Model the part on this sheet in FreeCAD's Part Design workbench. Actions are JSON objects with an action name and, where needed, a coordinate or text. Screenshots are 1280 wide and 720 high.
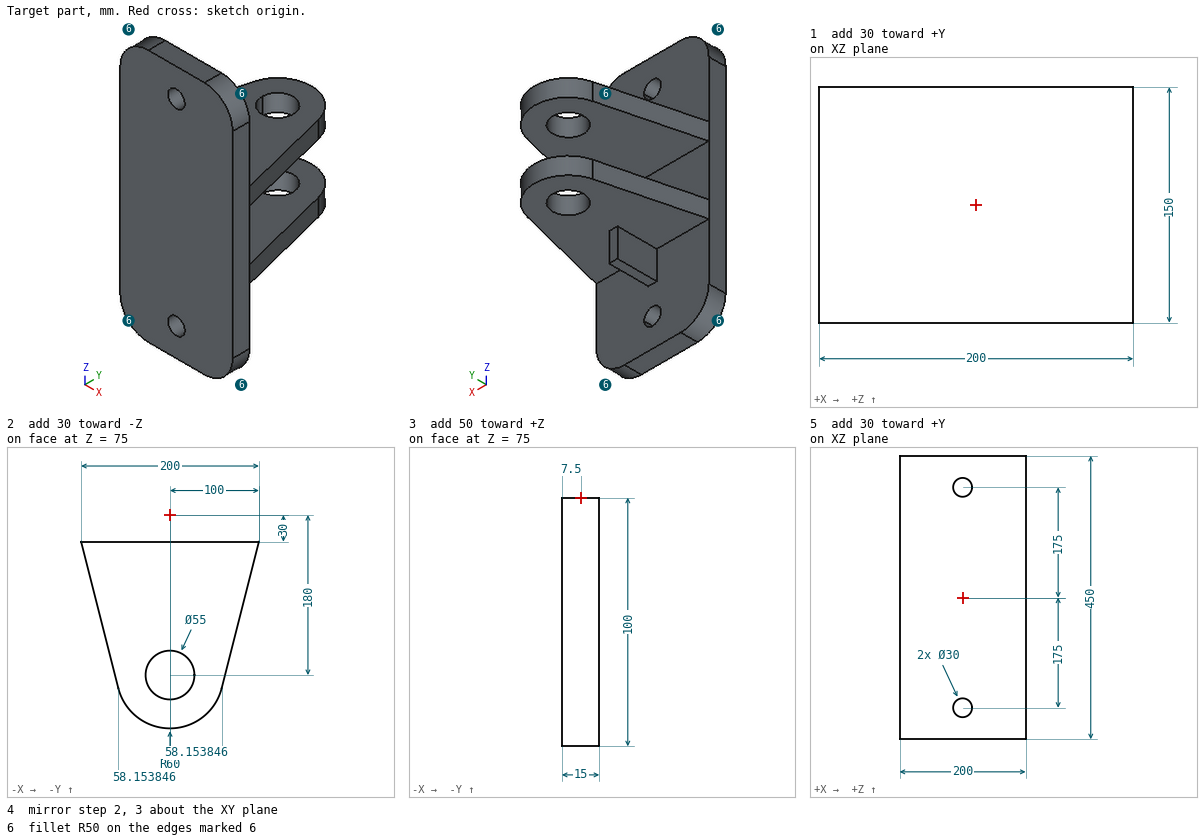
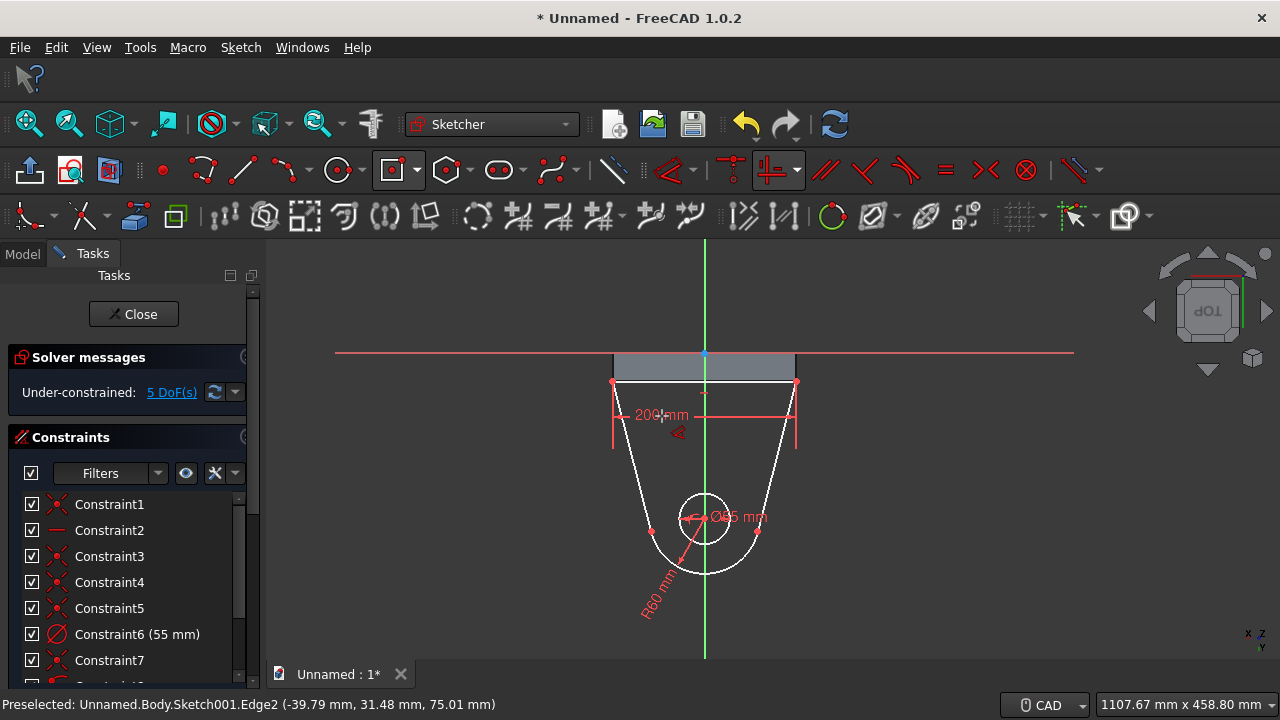
{"action": "scroll", "coordinate": [796, 382], "scroll_direction": "up", "scroll_amount": 2}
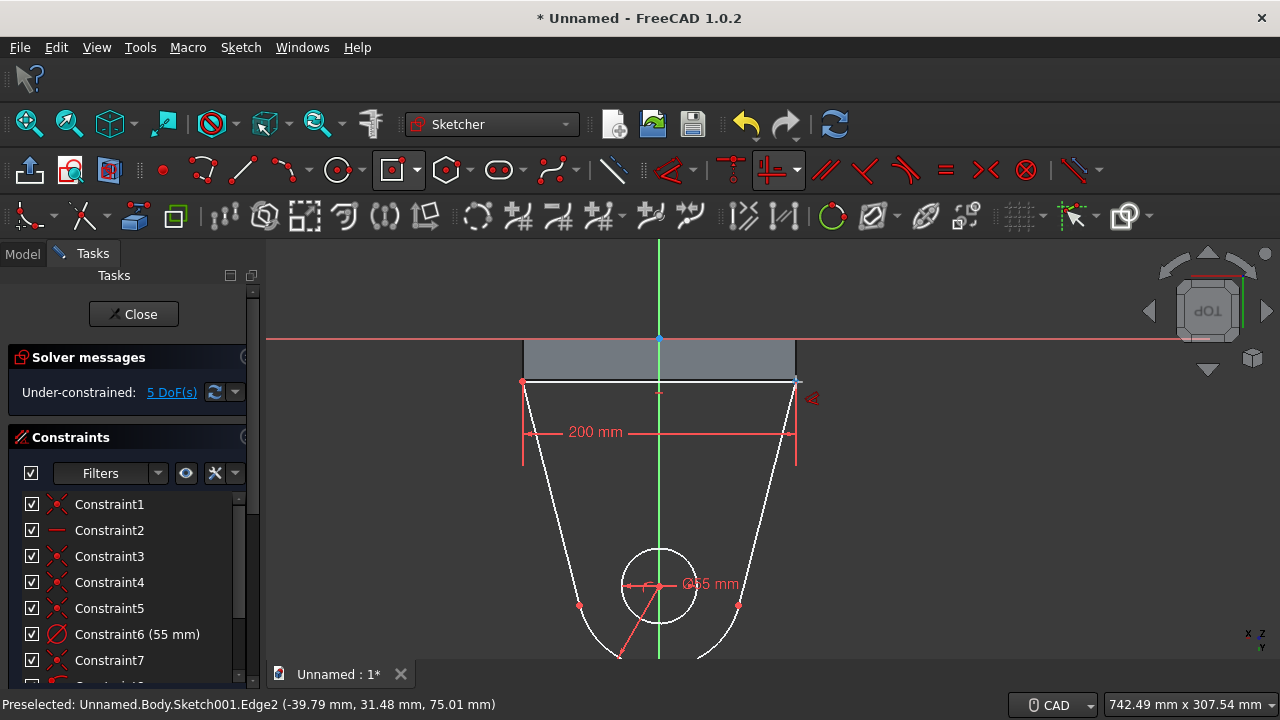
{"action": "left_click", "coordinate": [796, 382]}
{"action": "left_click", "coordinate": [830, 360]}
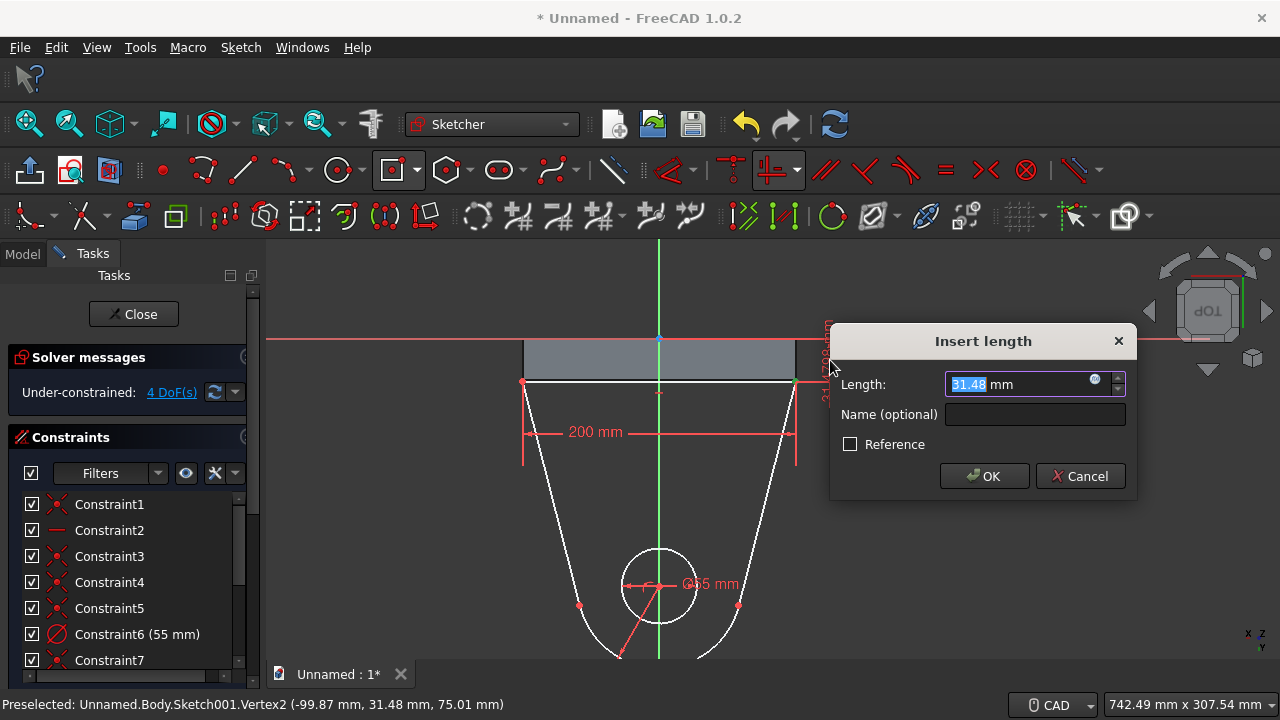
{"action": "type", "text": "30"}
{"action": "key", "text": "Return"}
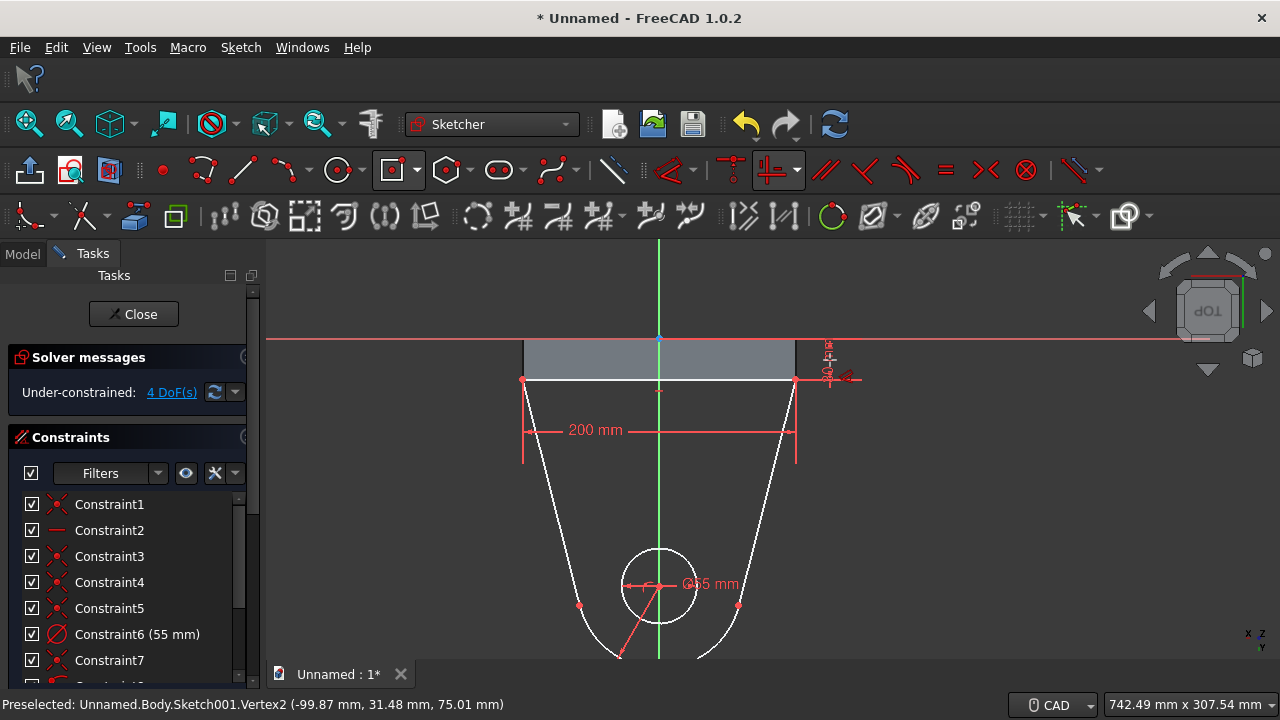
{"action": "left_click", "coordinate": [659, 586]}
{"action": "left_click", "coordinate": [693, 462]}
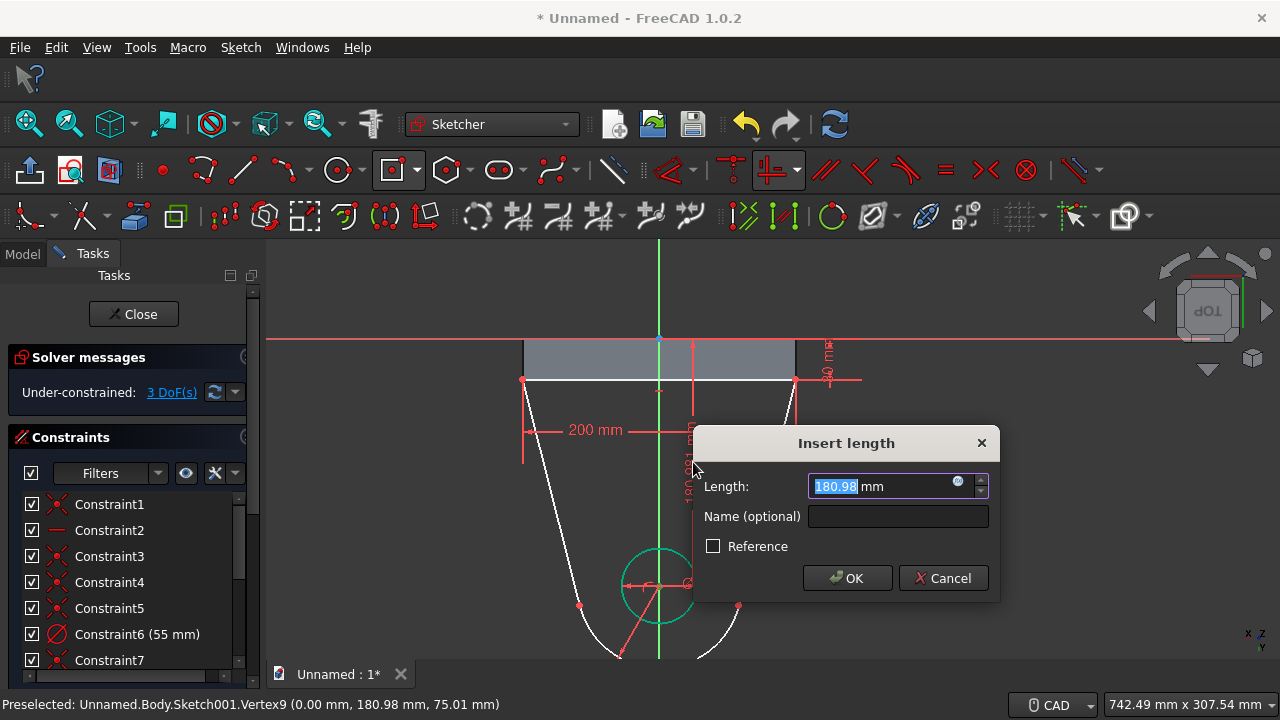
{"action": "type", "text": "180"}
{"action": "key", "text": "Return"}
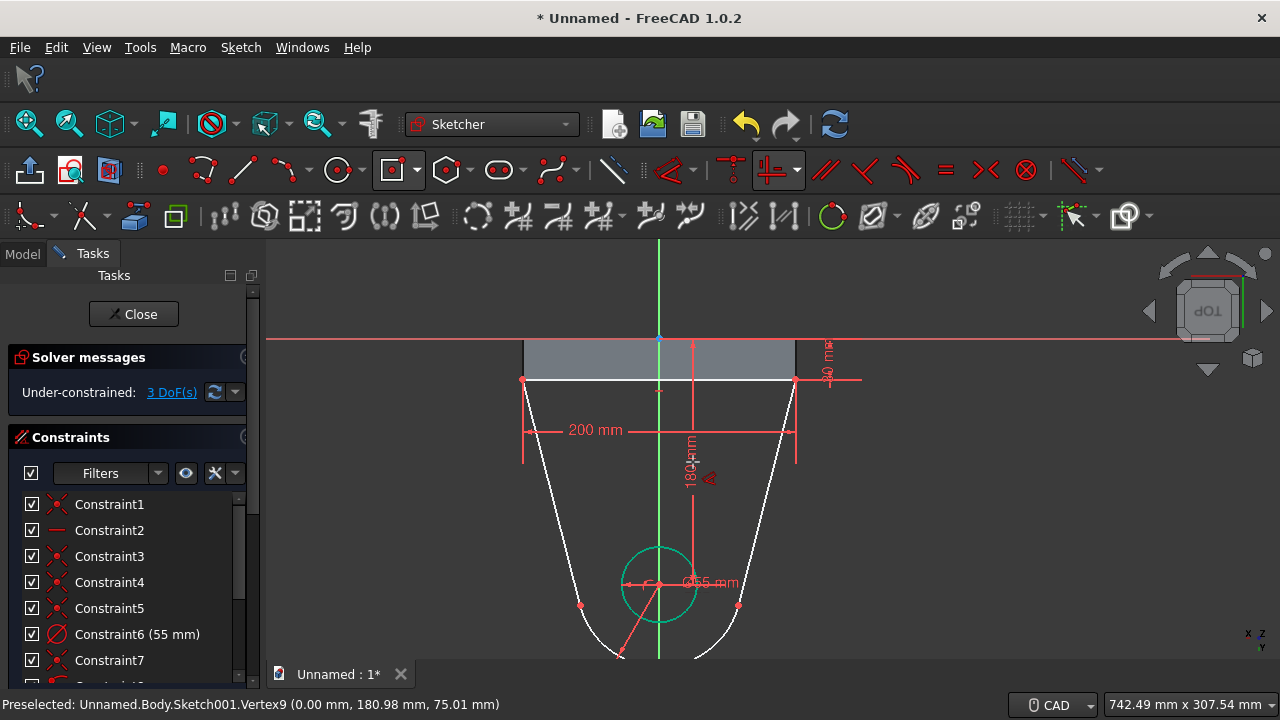
{"action": "left_click", "coordinate": [796, 380]}
{"action": "left_click", "coordinate": [728, 305]}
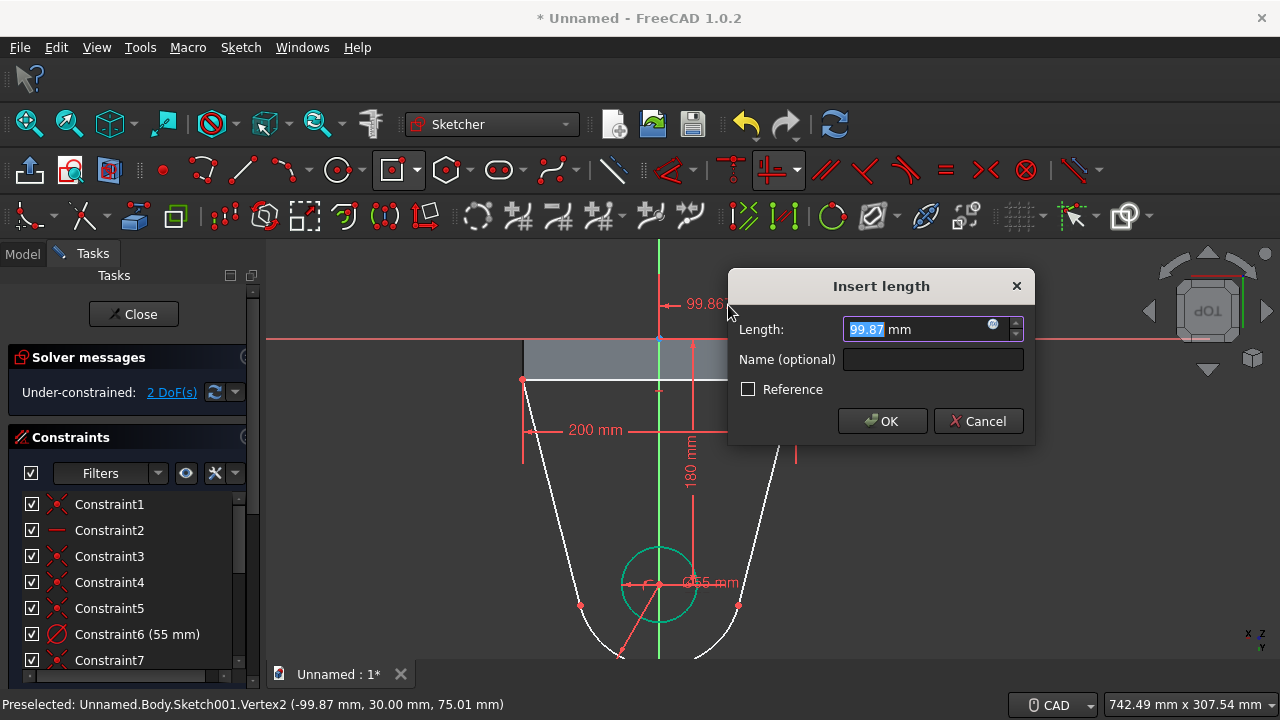
{"action": "type", "text": "100"}
{"action": "key", "text": "Return"}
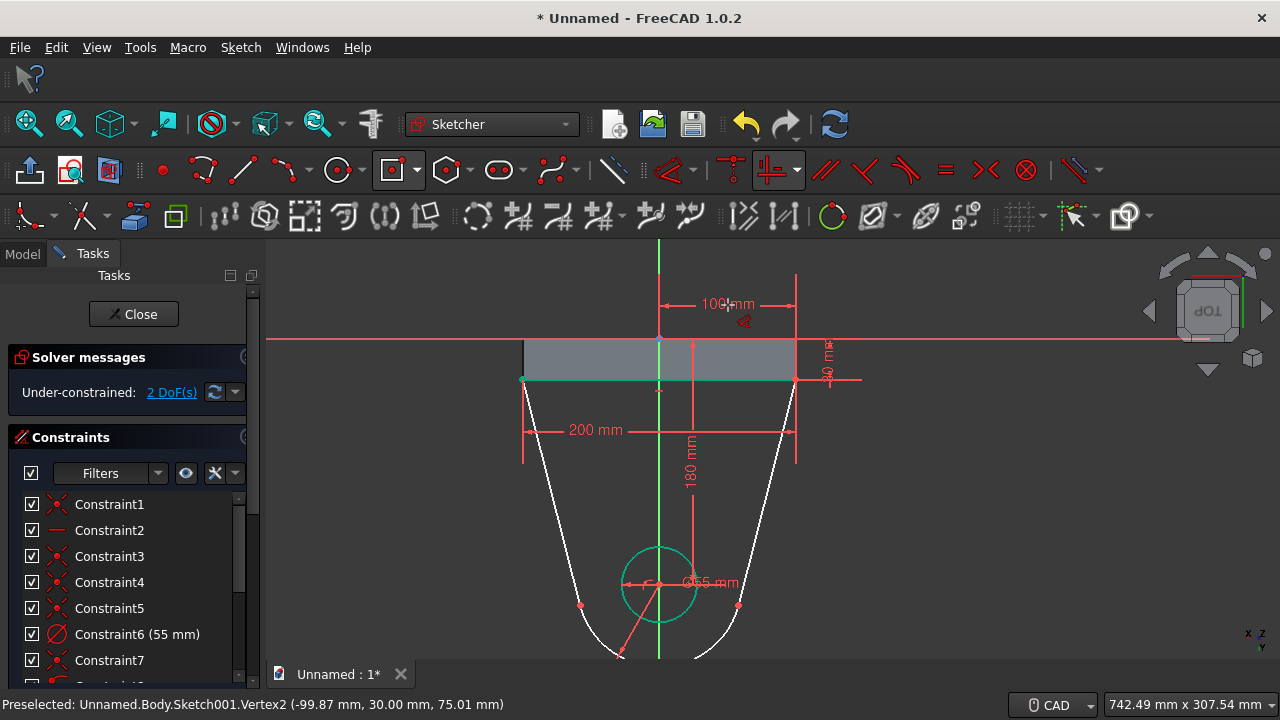
{"action": "left_click", "coordinate": [739, 606]}
{"action": "left_click", "coordinate": [699, 281]}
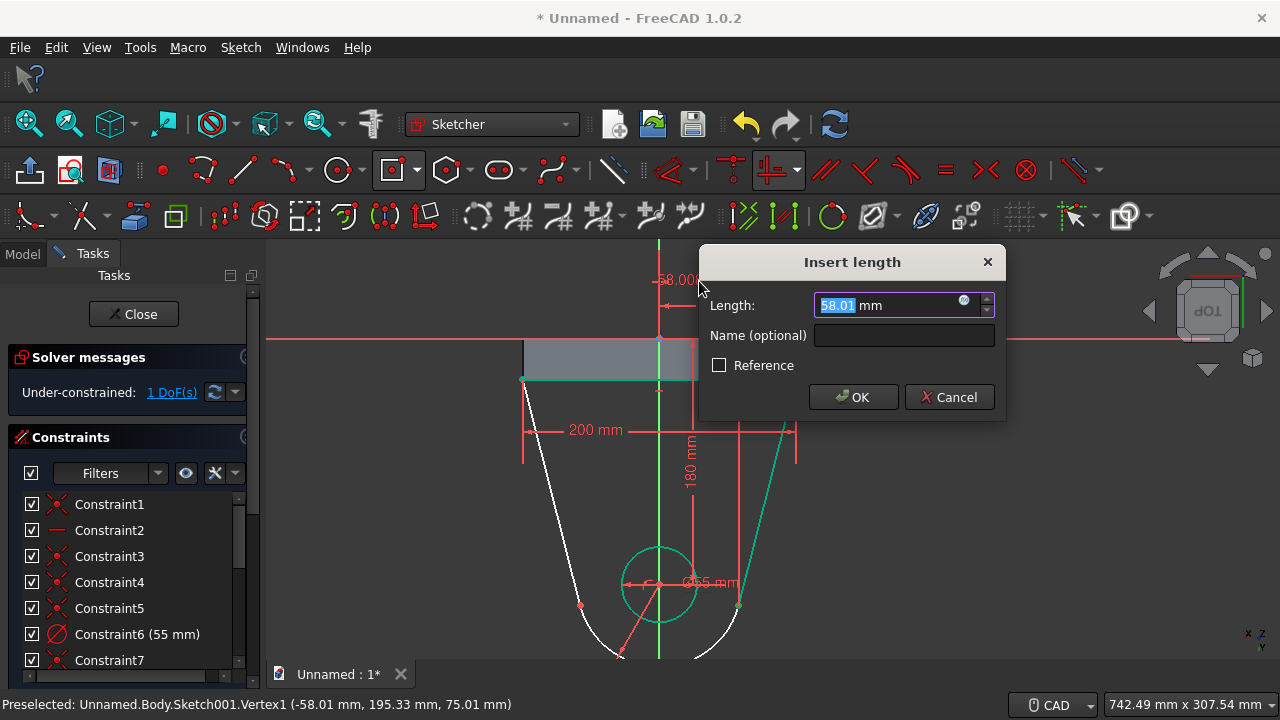
{"action": "type", "text": "58.153846"}
{"action": "key", "text": "Return"}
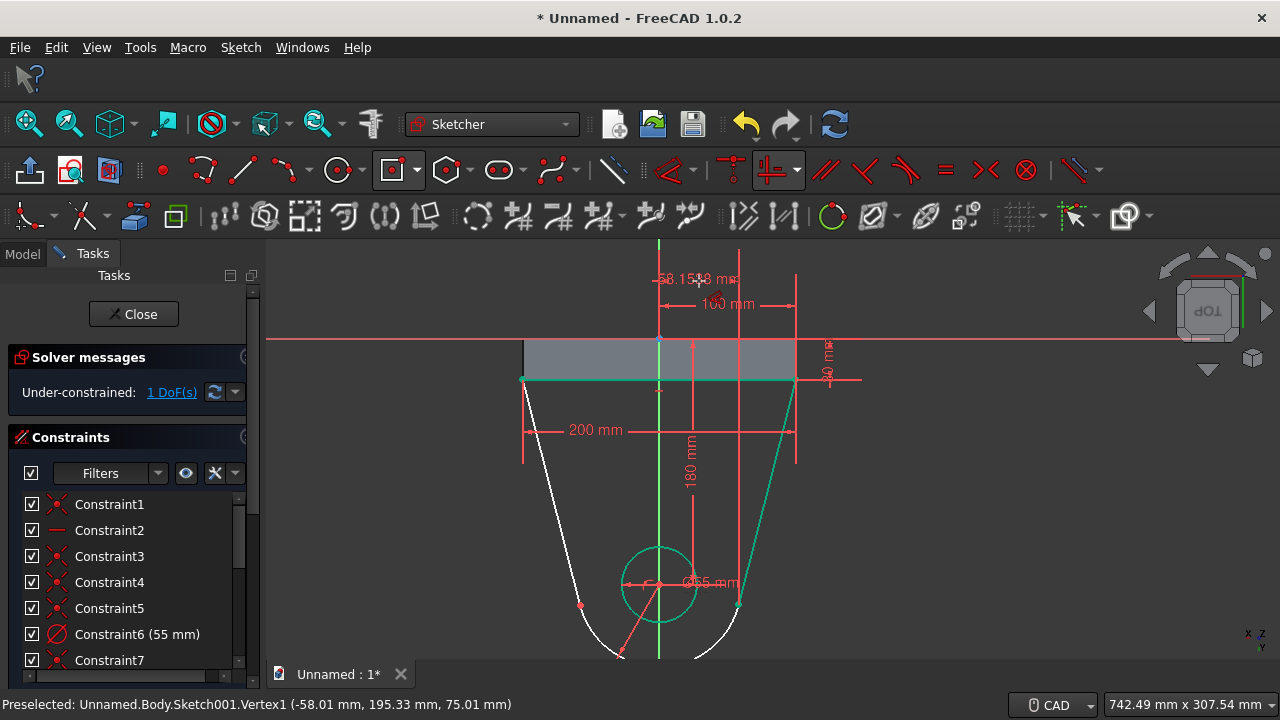
{"action": "left_click", "coordinate": [580, 606]}
{"action": "left_click", "coordinate": [620, 305]}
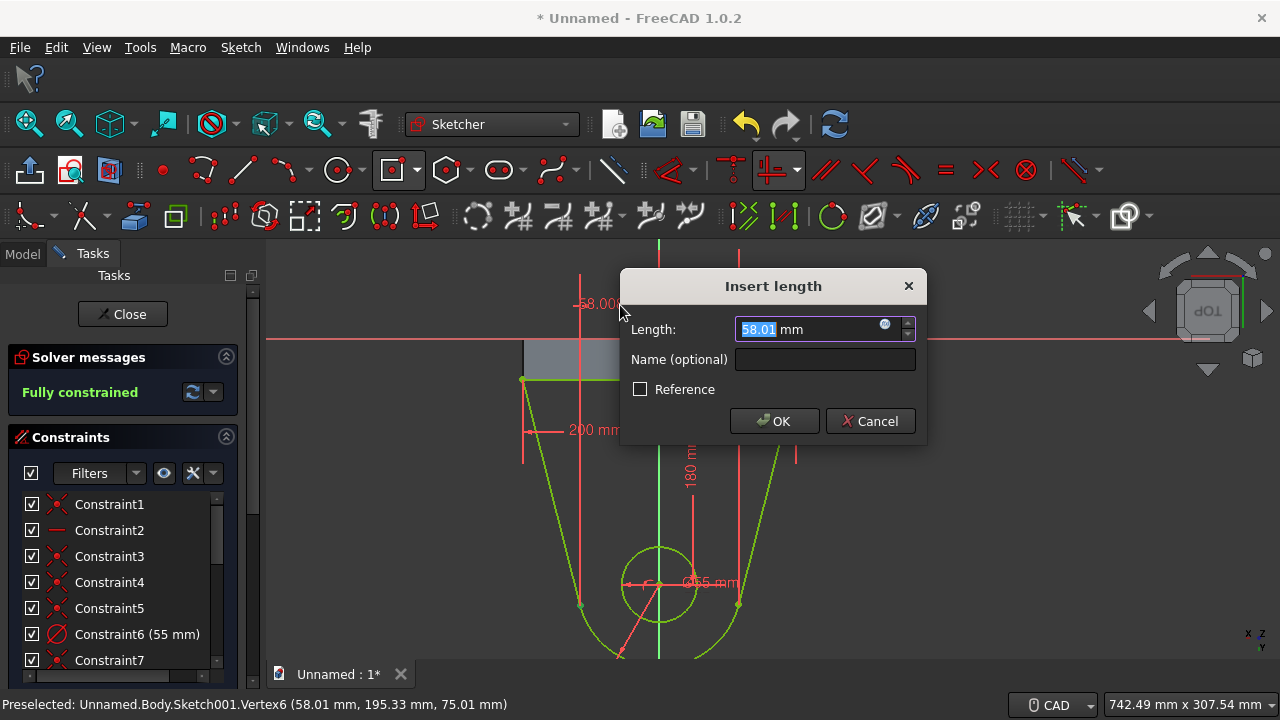
{"action": "type", "text": "58.153846"}
{"action": "key", "text": "Return"}
{"action": "key", "text": "Escape"}